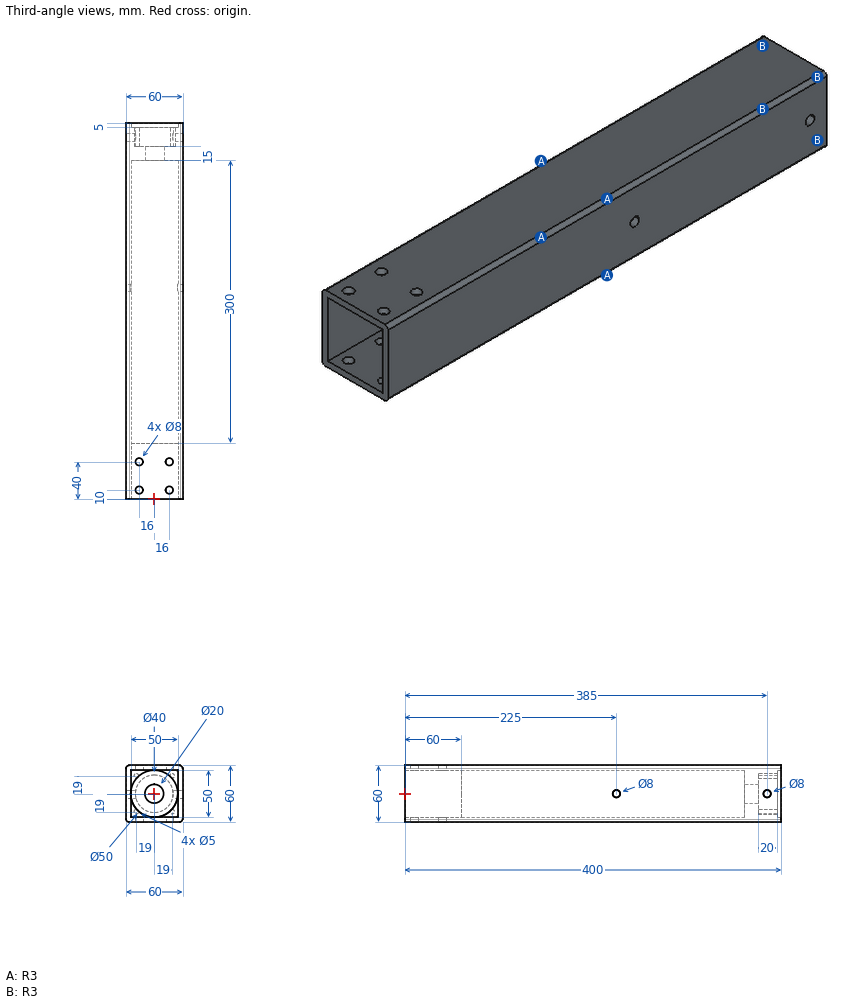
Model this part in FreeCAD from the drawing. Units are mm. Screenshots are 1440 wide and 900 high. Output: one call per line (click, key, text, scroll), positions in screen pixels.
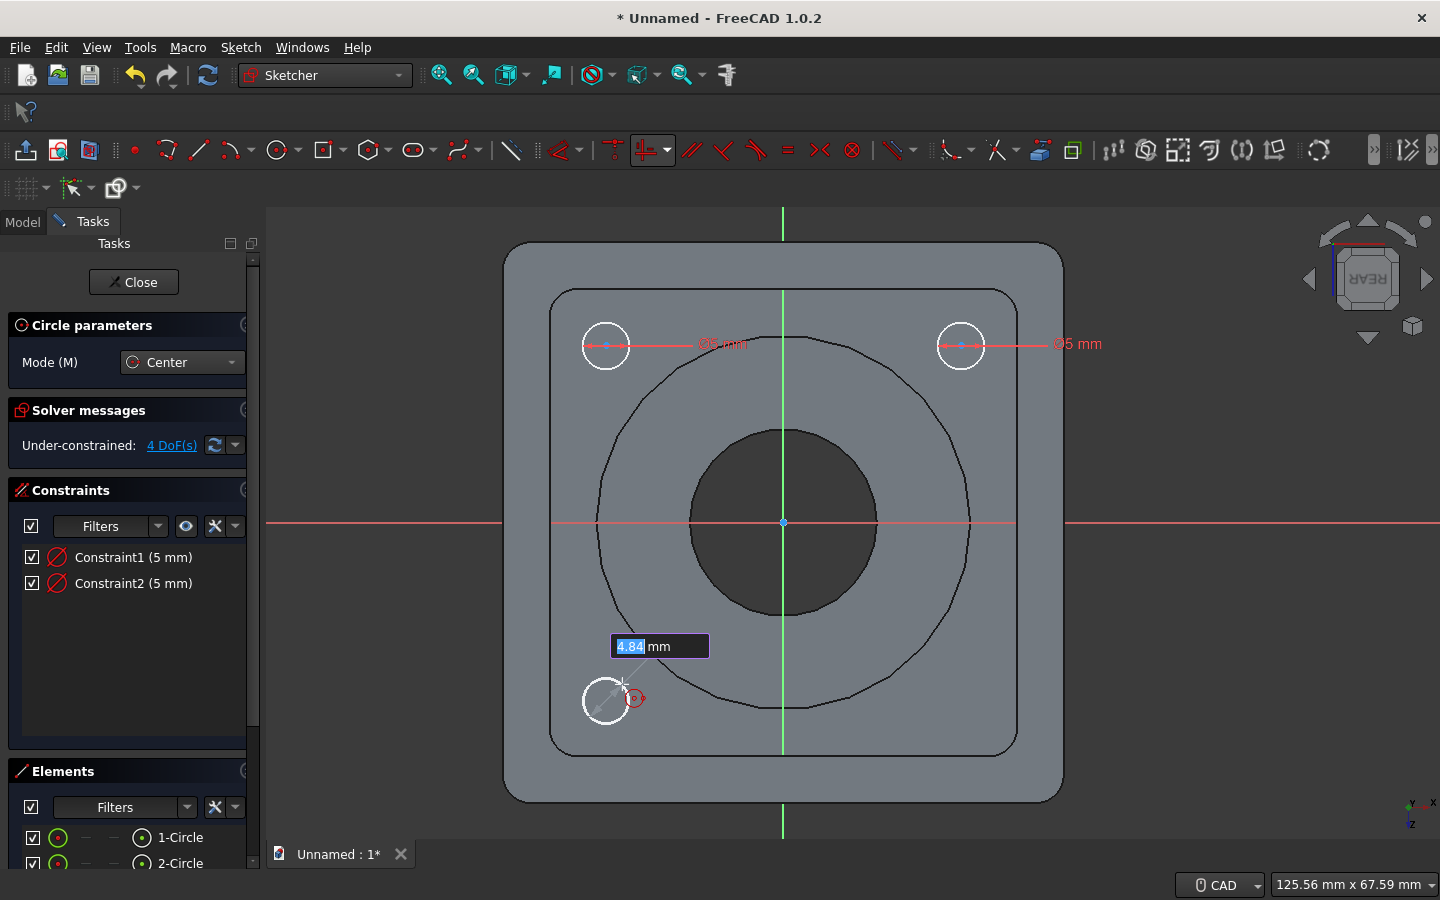
text(5)
key(Return)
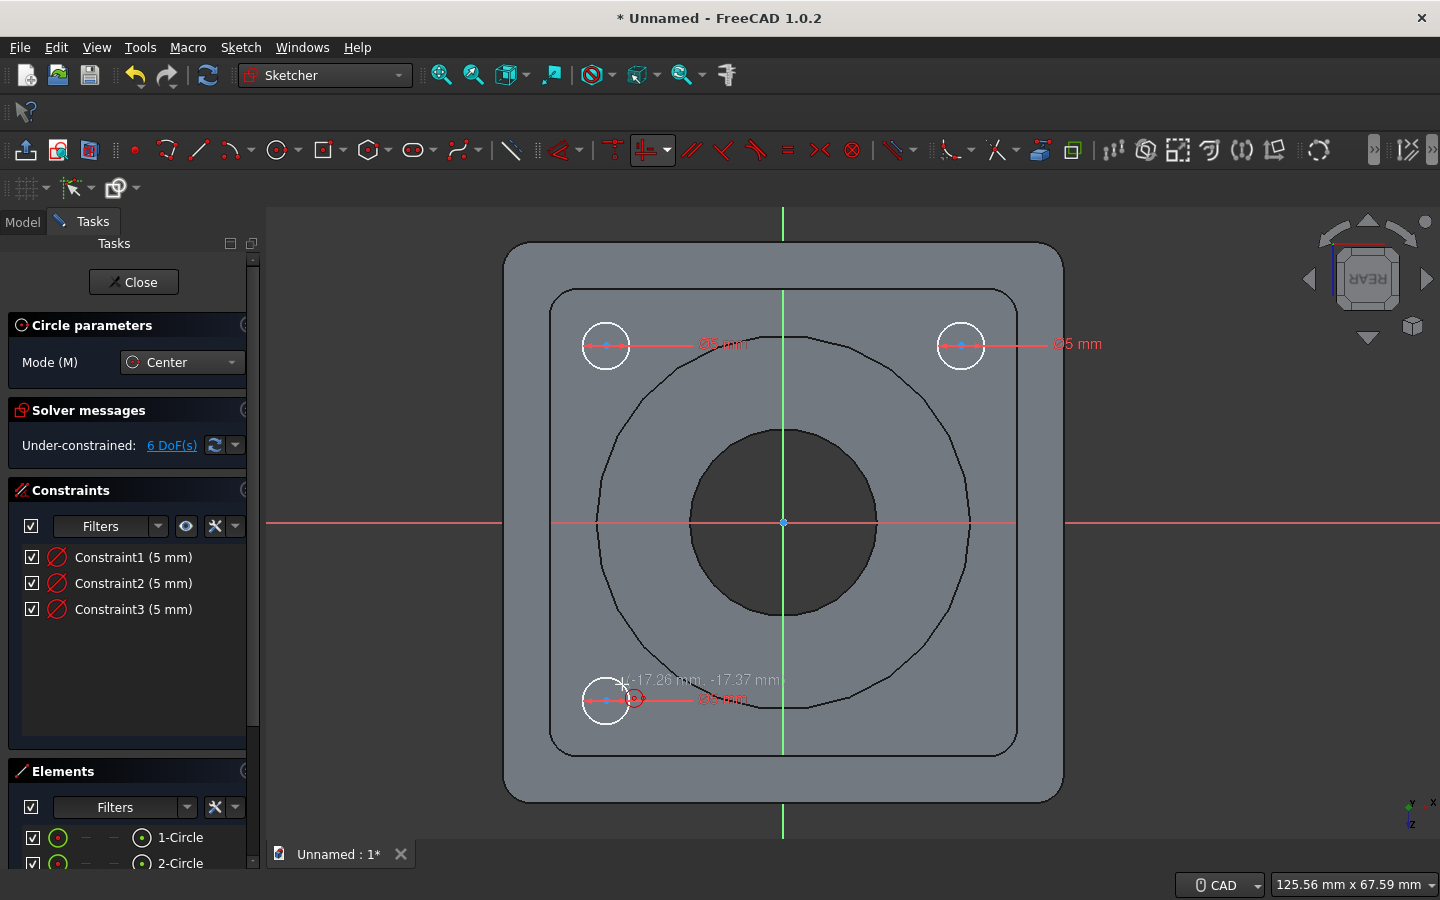
click(961, 700)
move(978, 684)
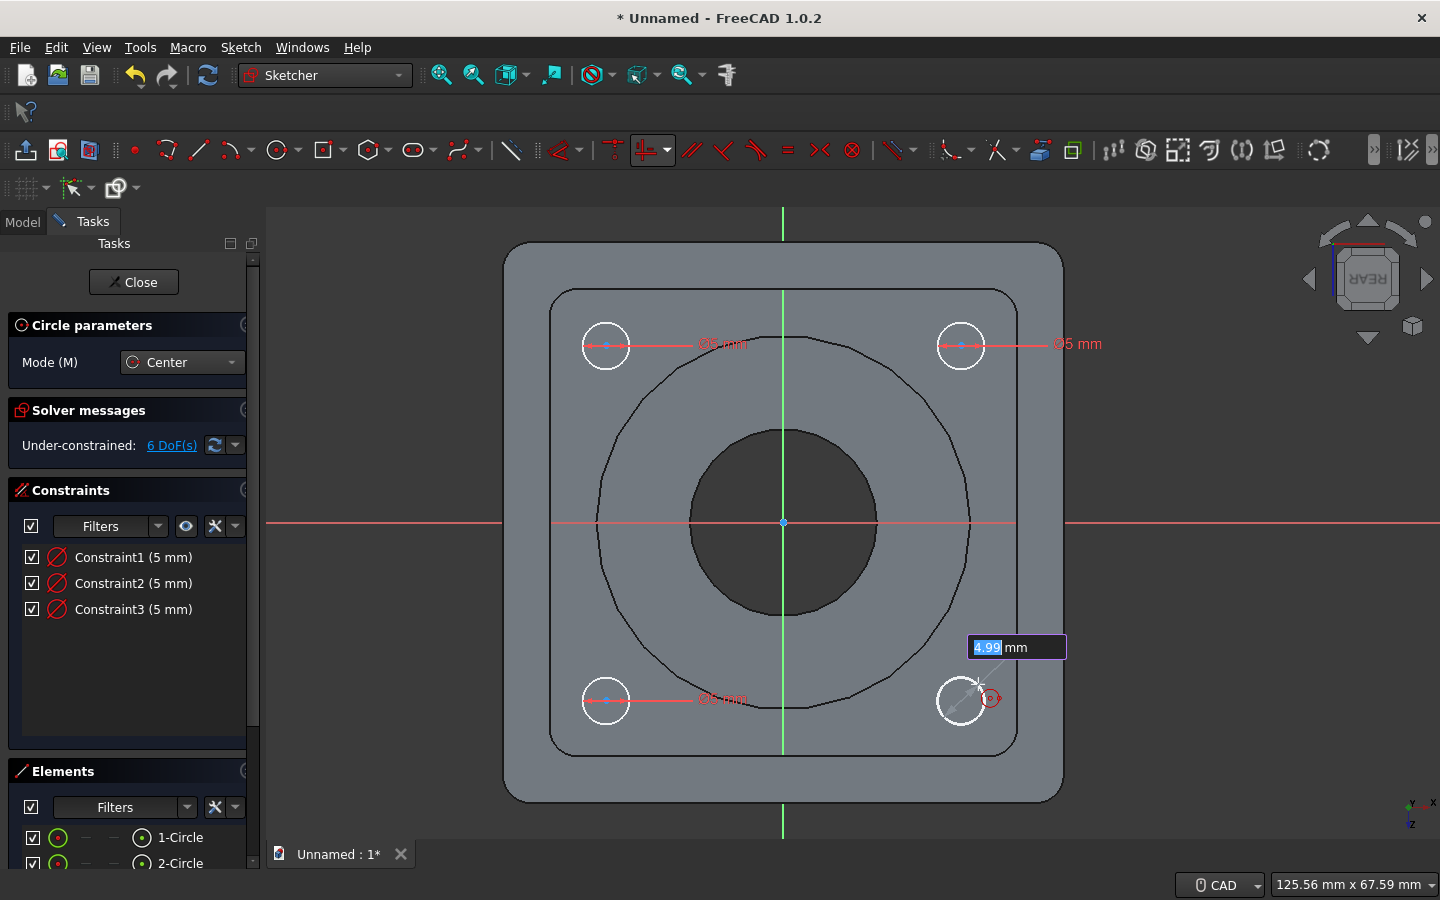
text(5)
key(Return)
key(Escape)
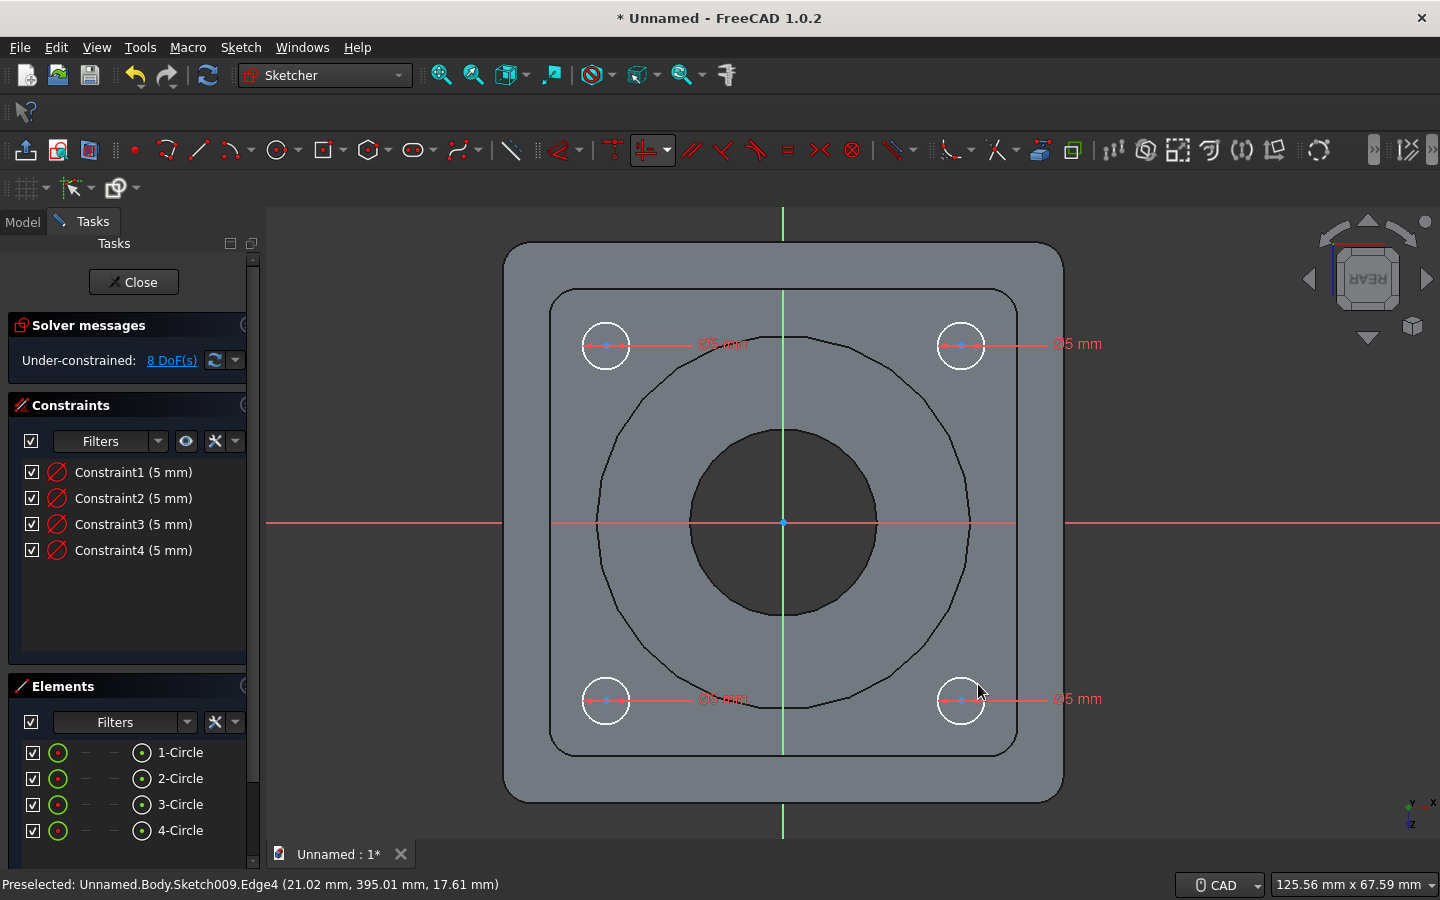
click(606, 346)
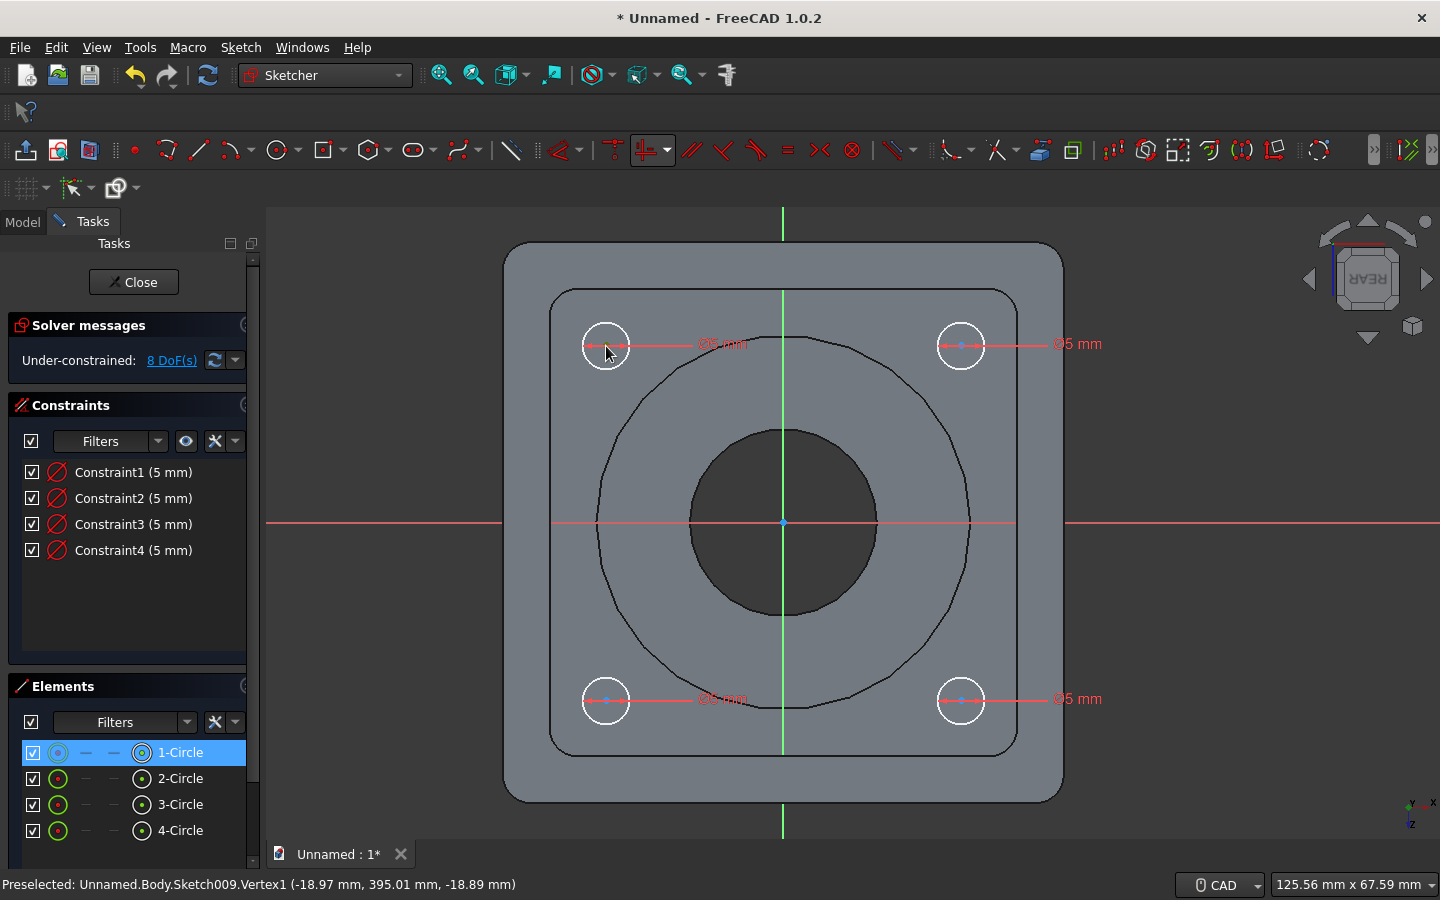
click(961, 346)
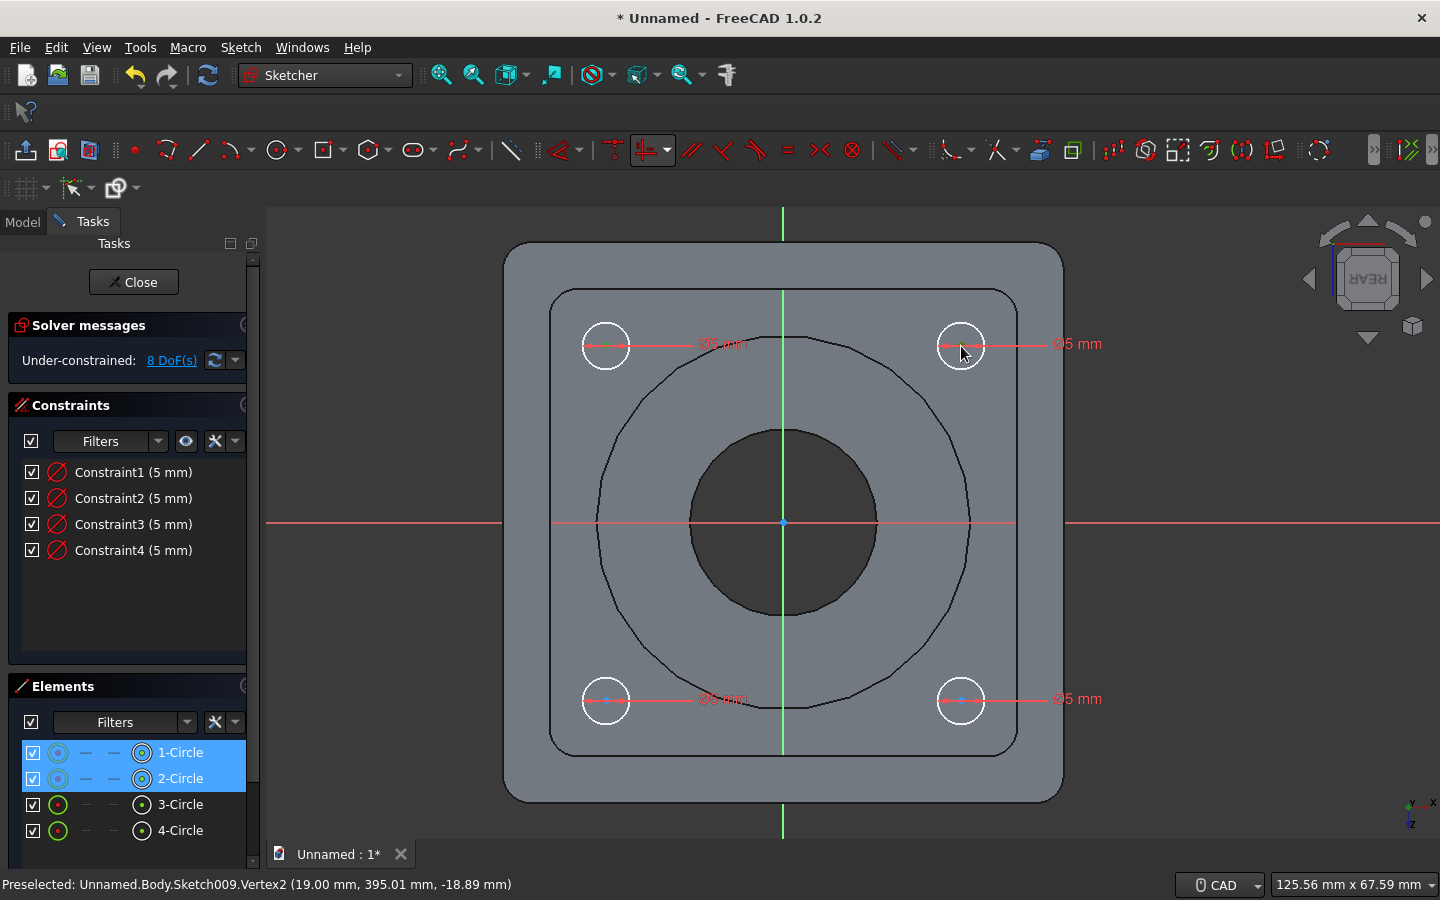
click(670, 150)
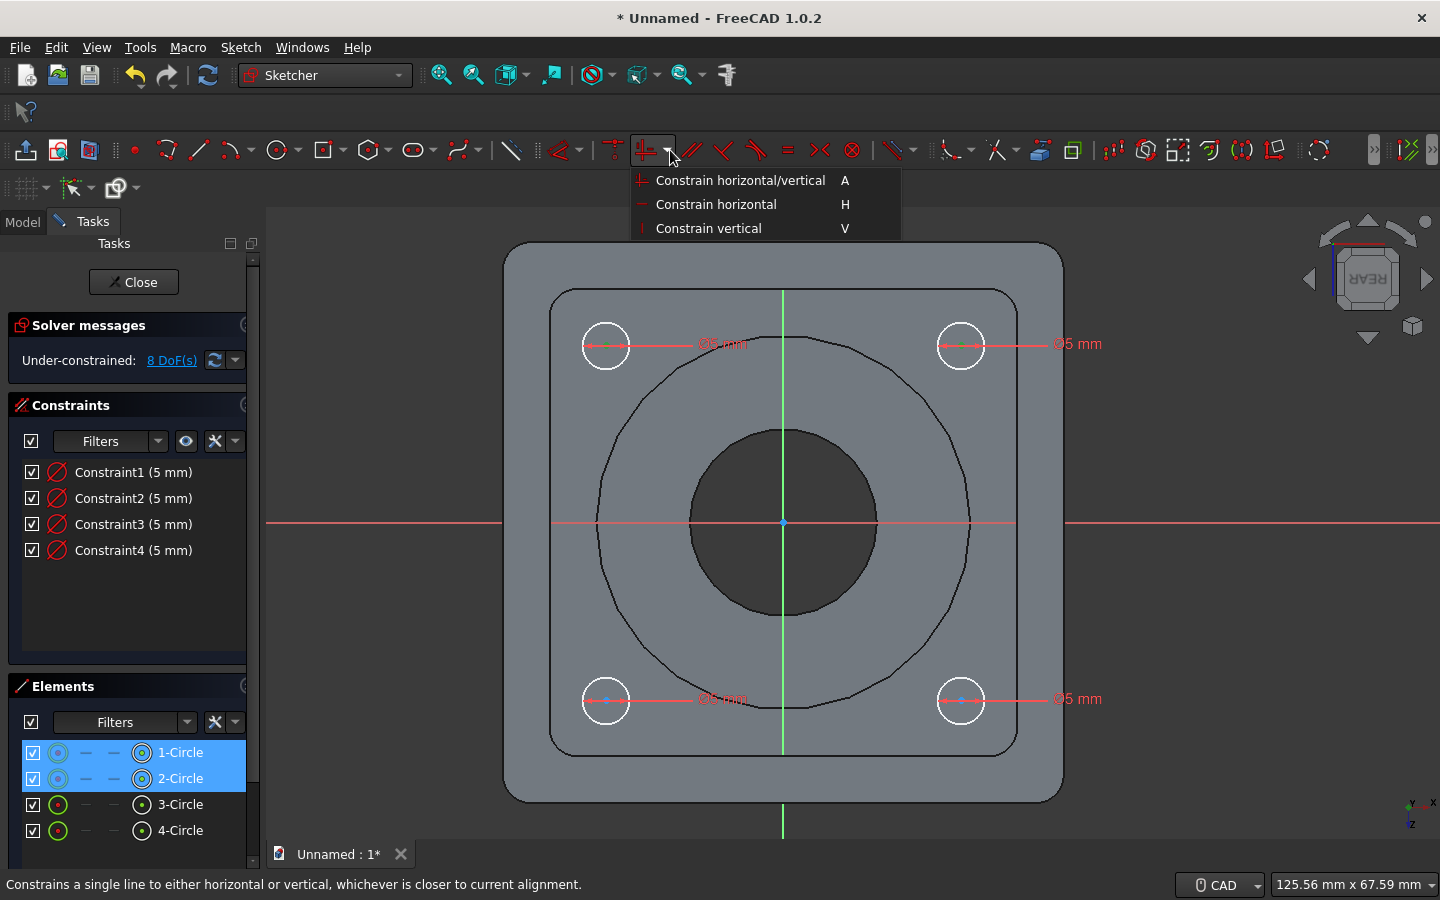
click(766, 204)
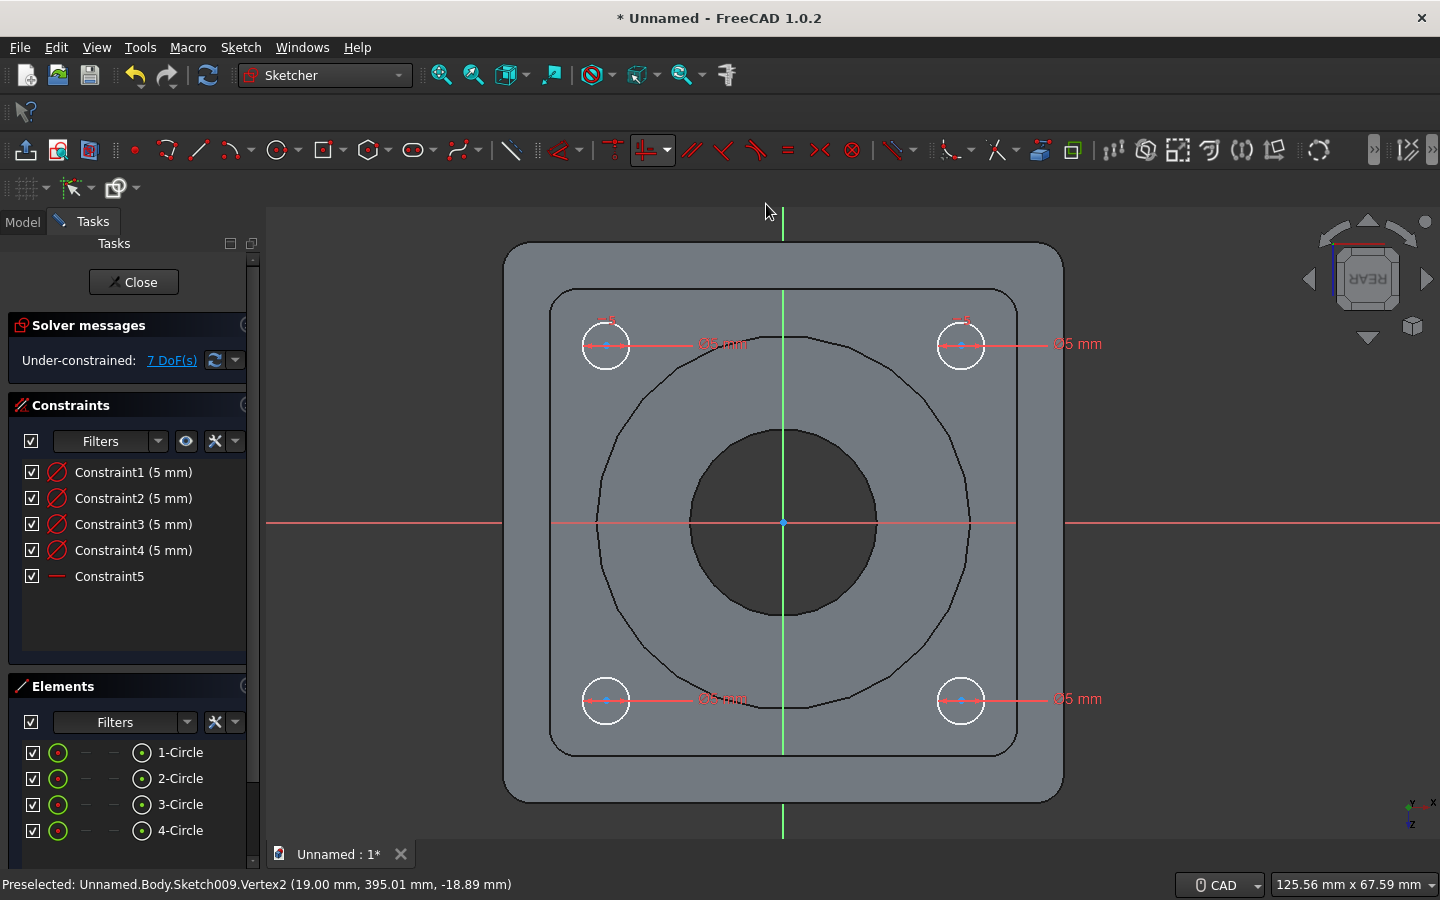
click(606, 346)